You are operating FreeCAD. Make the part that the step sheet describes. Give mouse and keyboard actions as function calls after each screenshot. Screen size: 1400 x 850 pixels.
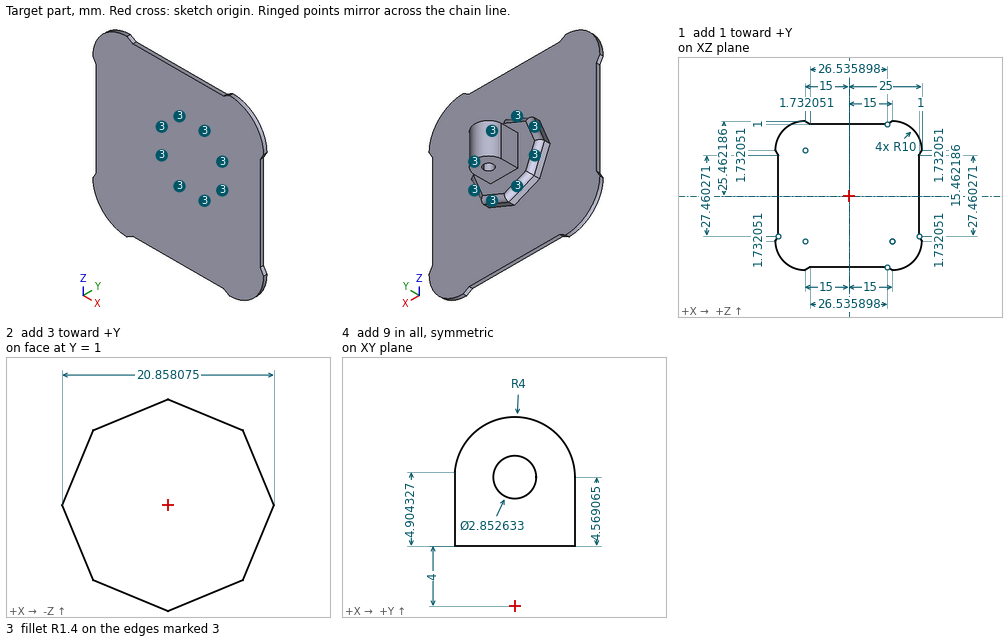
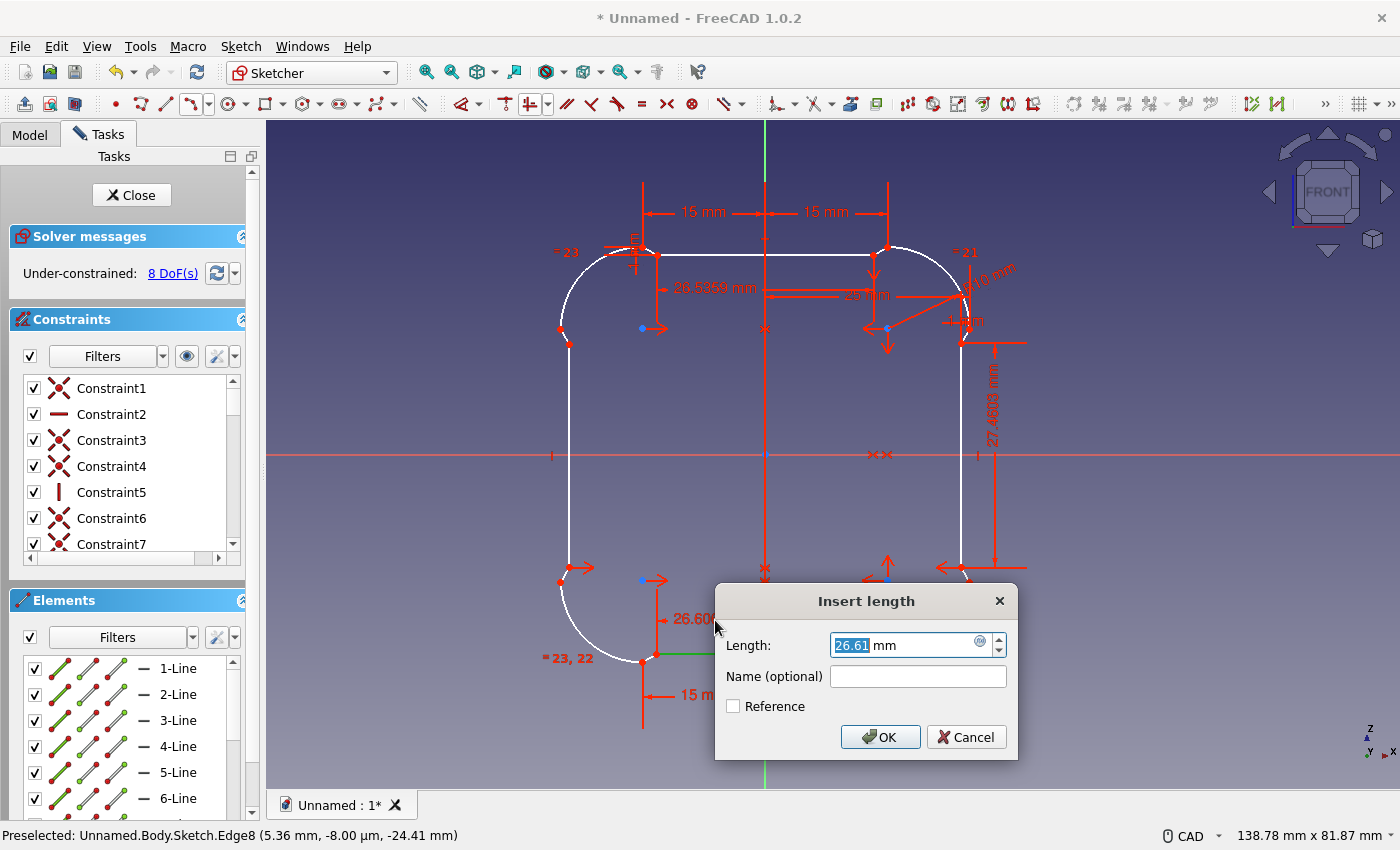
text(26.535898)
key(Return)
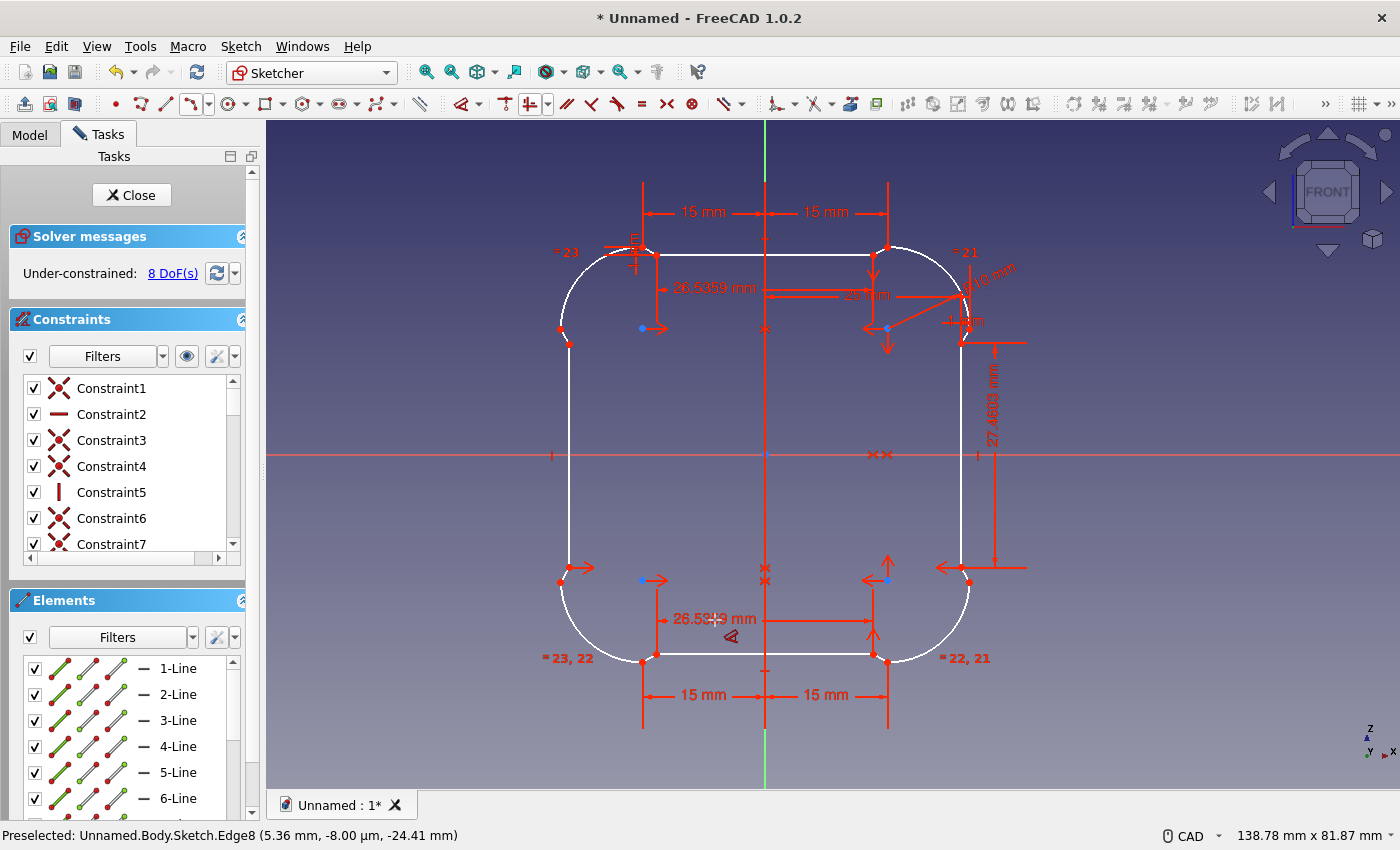
click(569, 501)
click(535, 405)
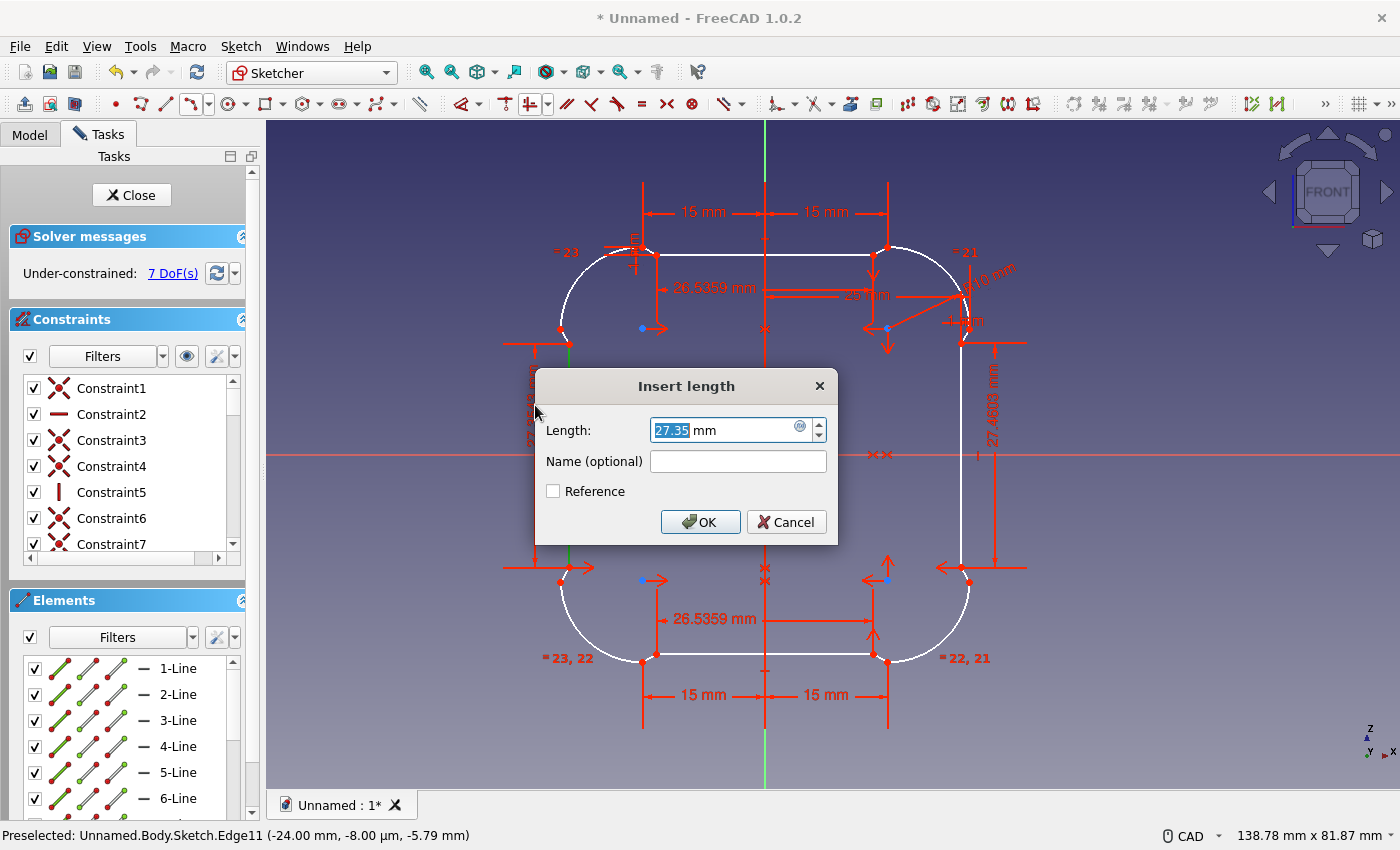
text(27.460271)
key(Return)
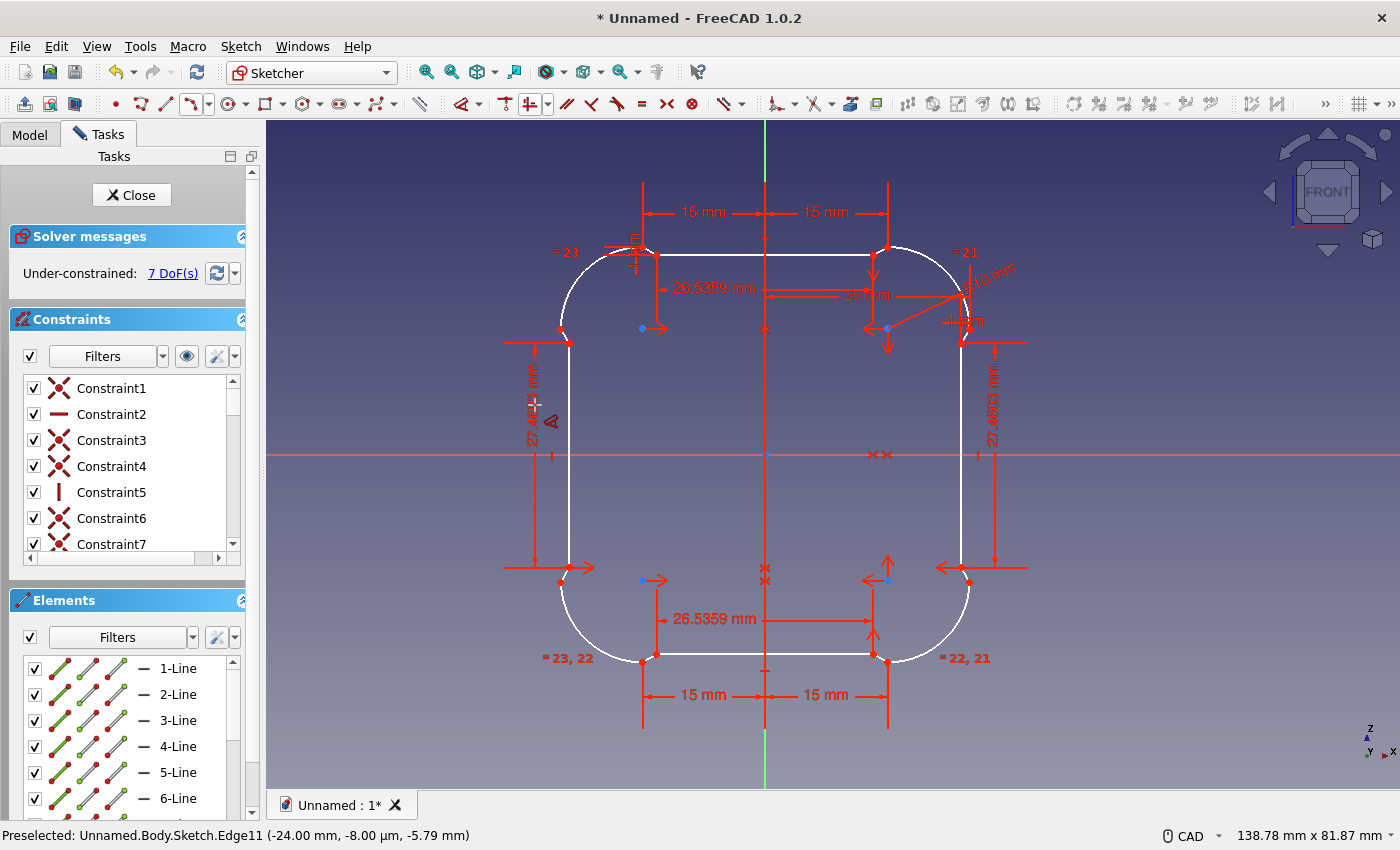
scroll(650, 251, up, 6)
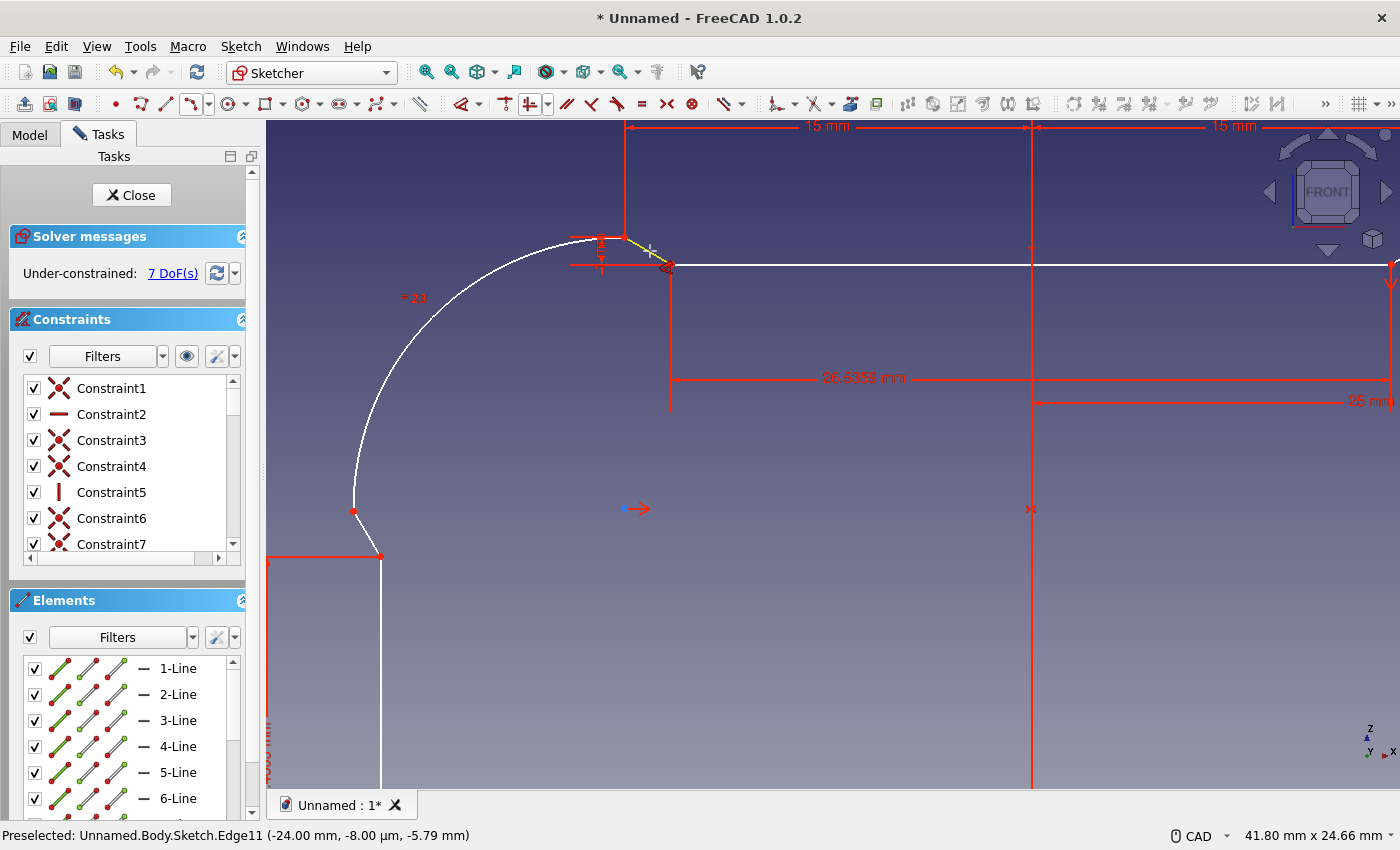
click(648, 251)
click(648, 203)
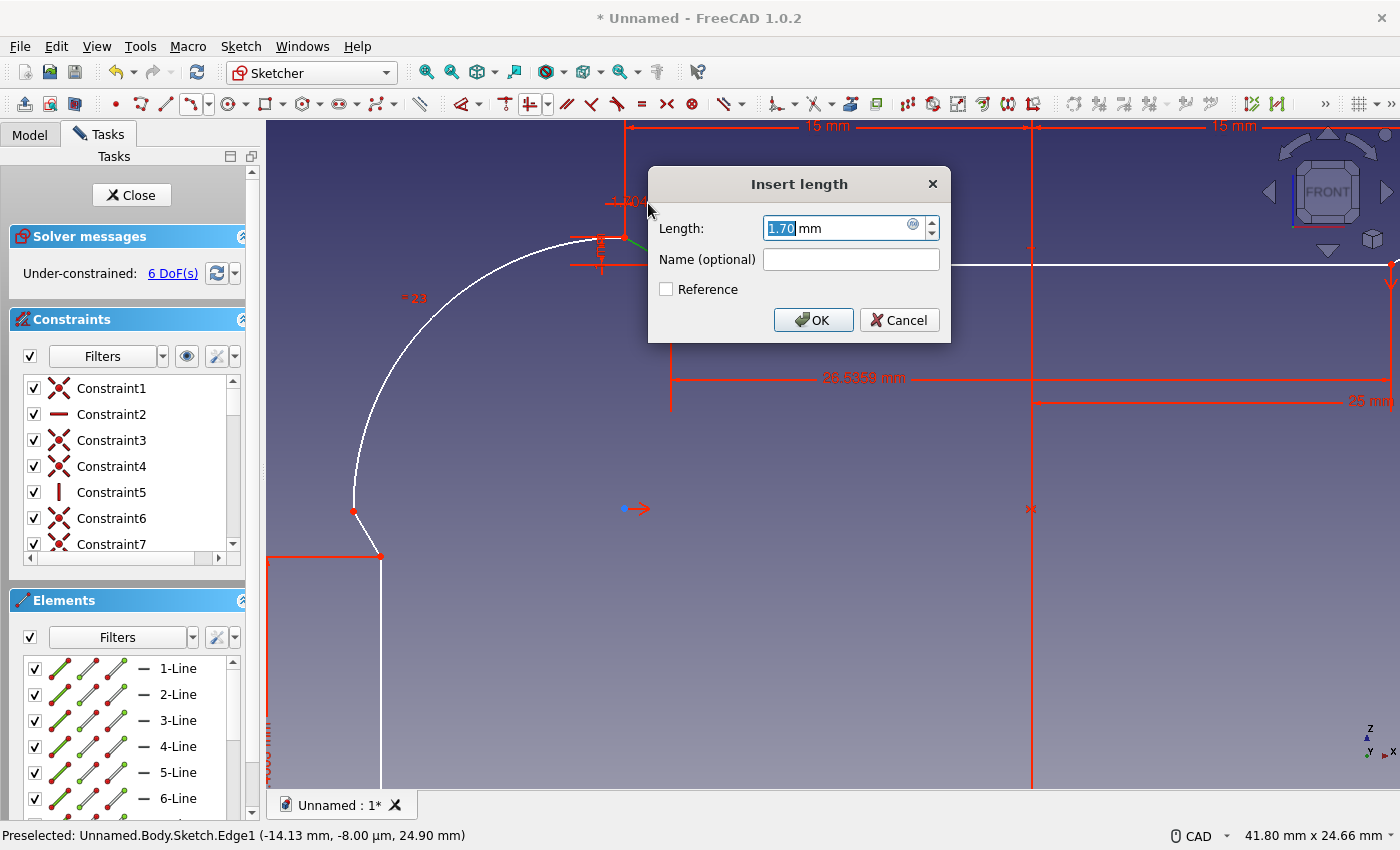
text(1.732051)
key(Return)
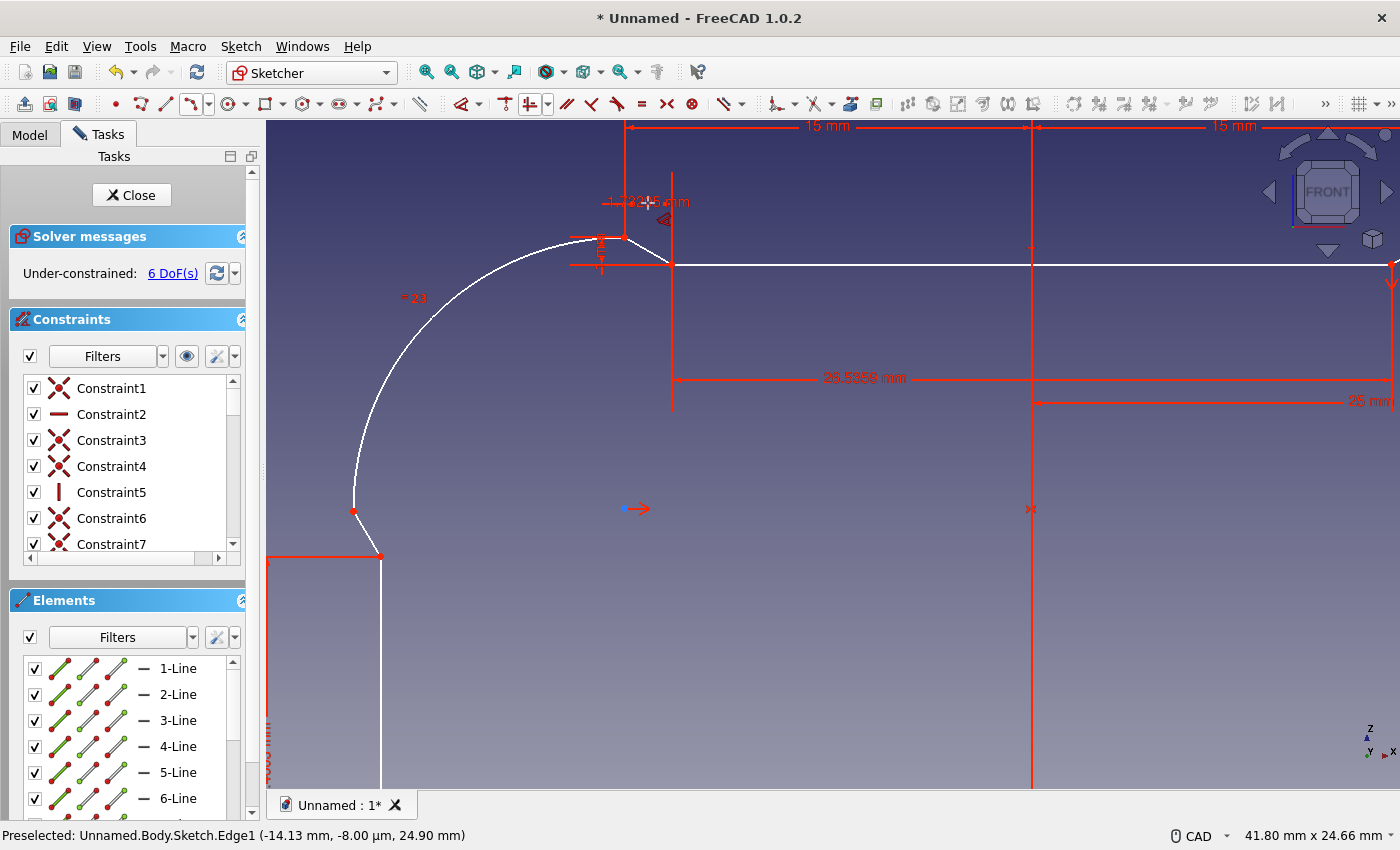
scroll(649, 251, down, 6)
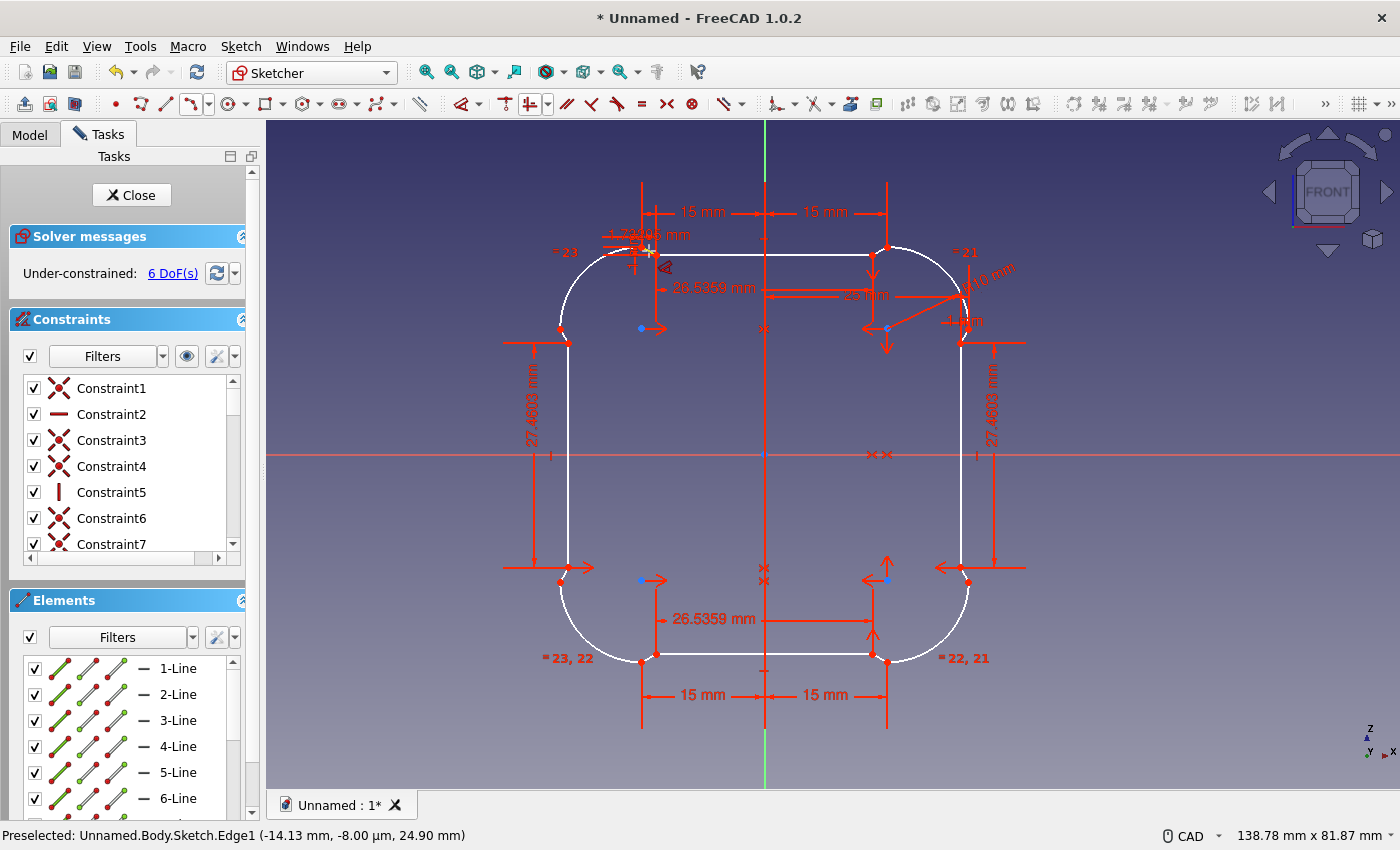
scroll(966, 334, up, 6)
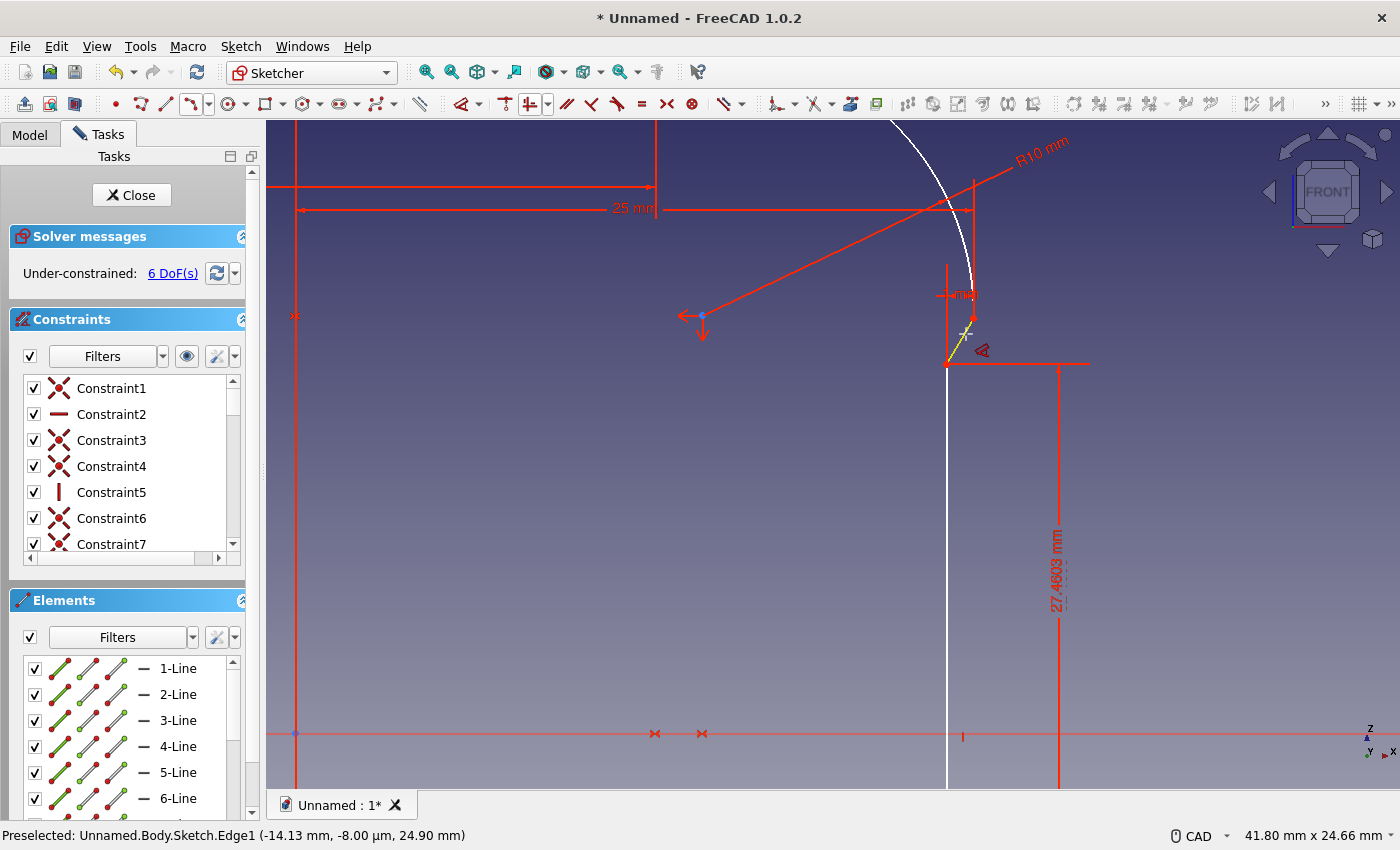
click(966, 332)
click(1008, 341)